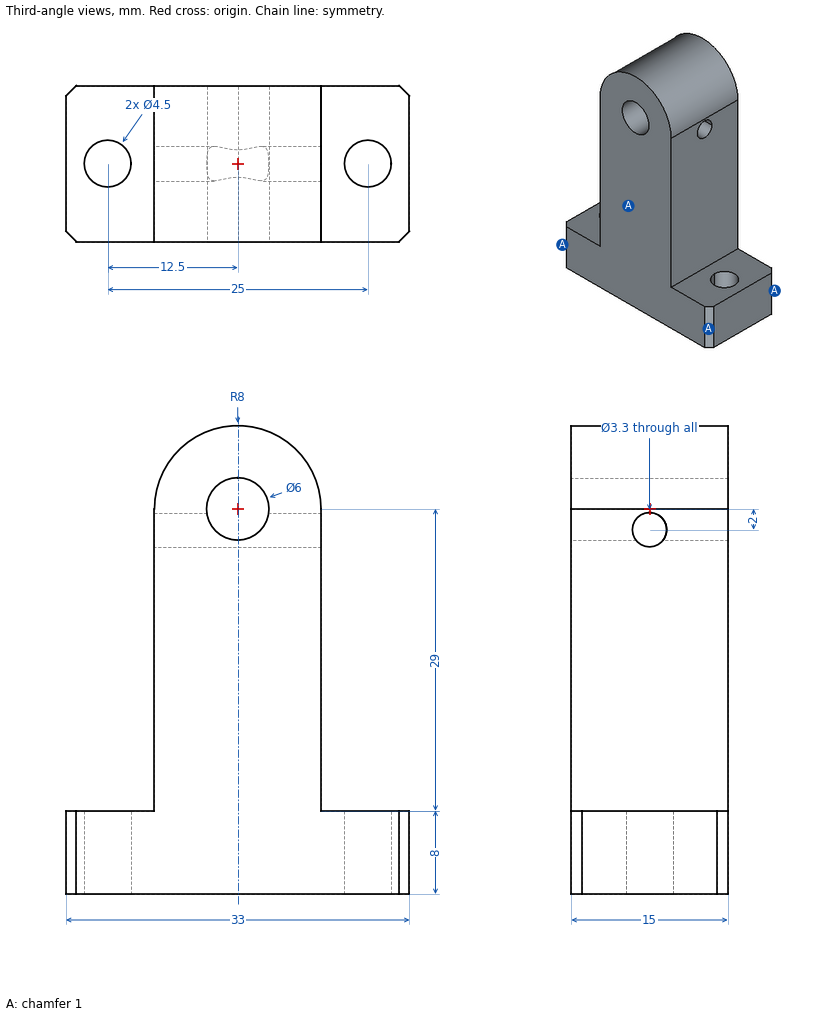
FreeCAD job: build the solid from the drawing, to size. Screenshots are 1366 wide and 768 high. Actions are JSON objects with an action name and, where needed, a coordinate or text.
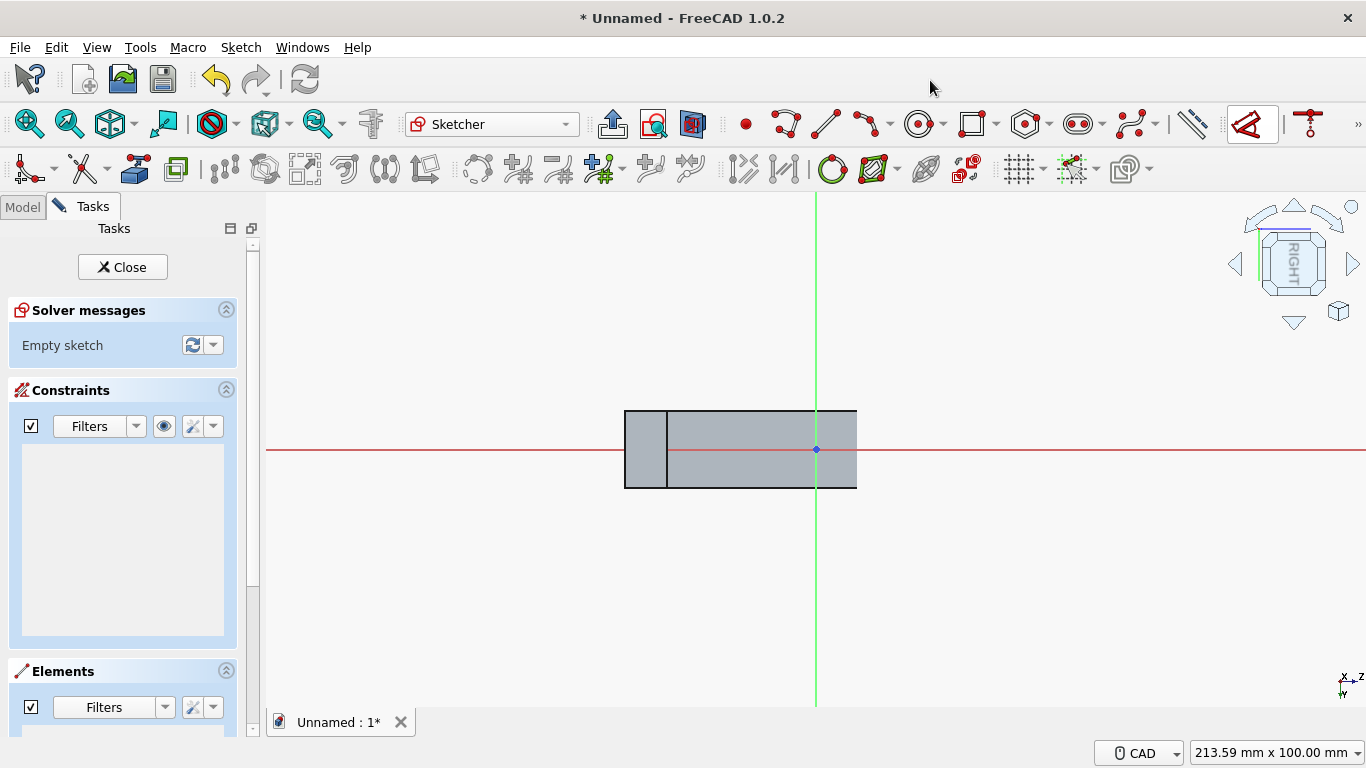
{"action": "left_click", "coordinate": [694, 124]}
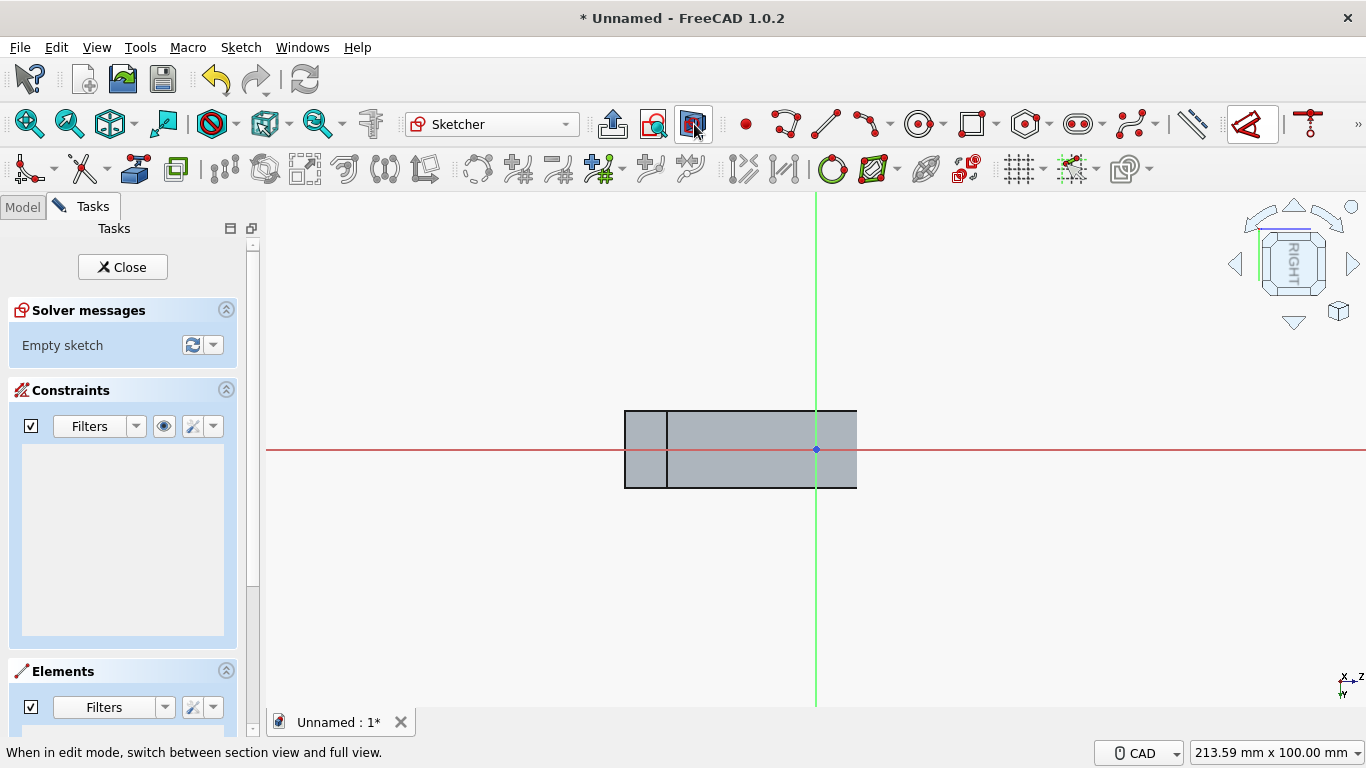
{"action": "scroll", "coordinate": [810, 450], "scroll_direction": "up", "scroll_amount": 15}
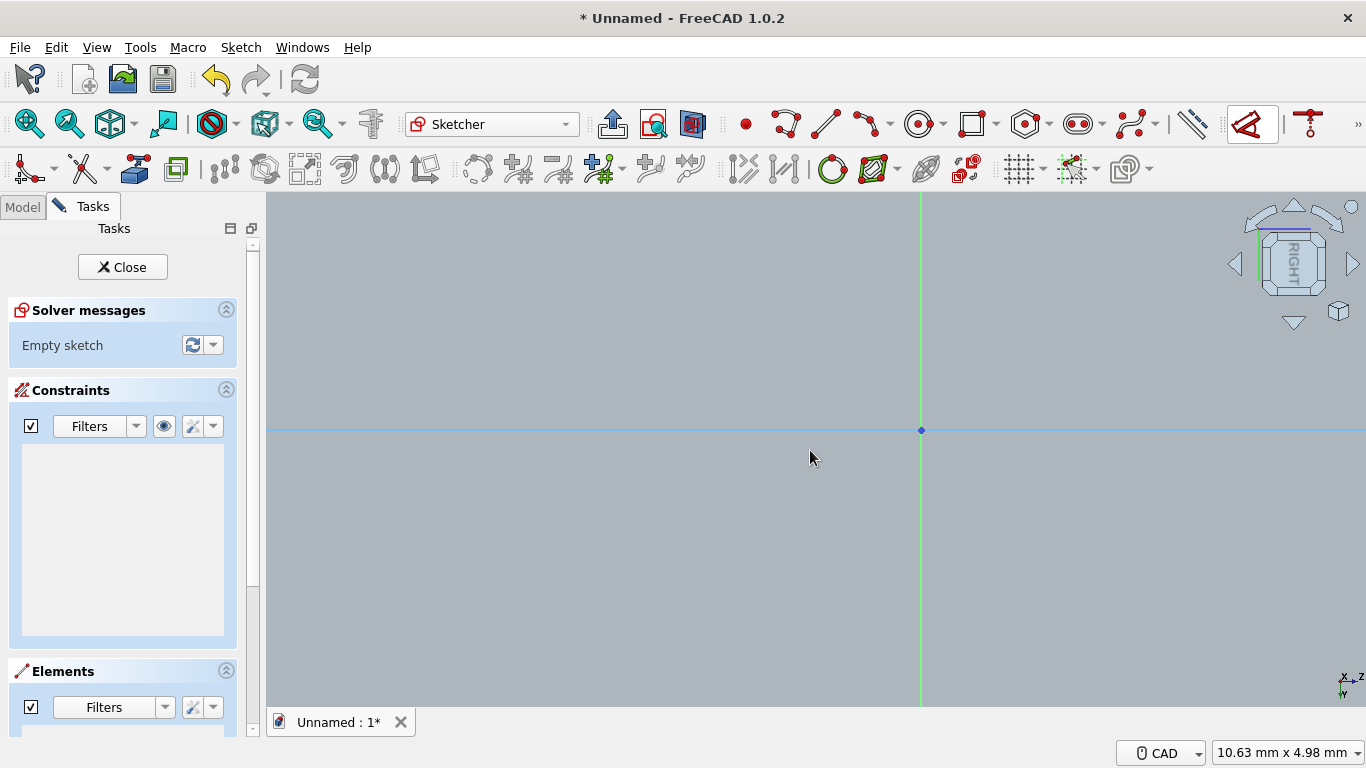
{"action": "key", "text": "g c"}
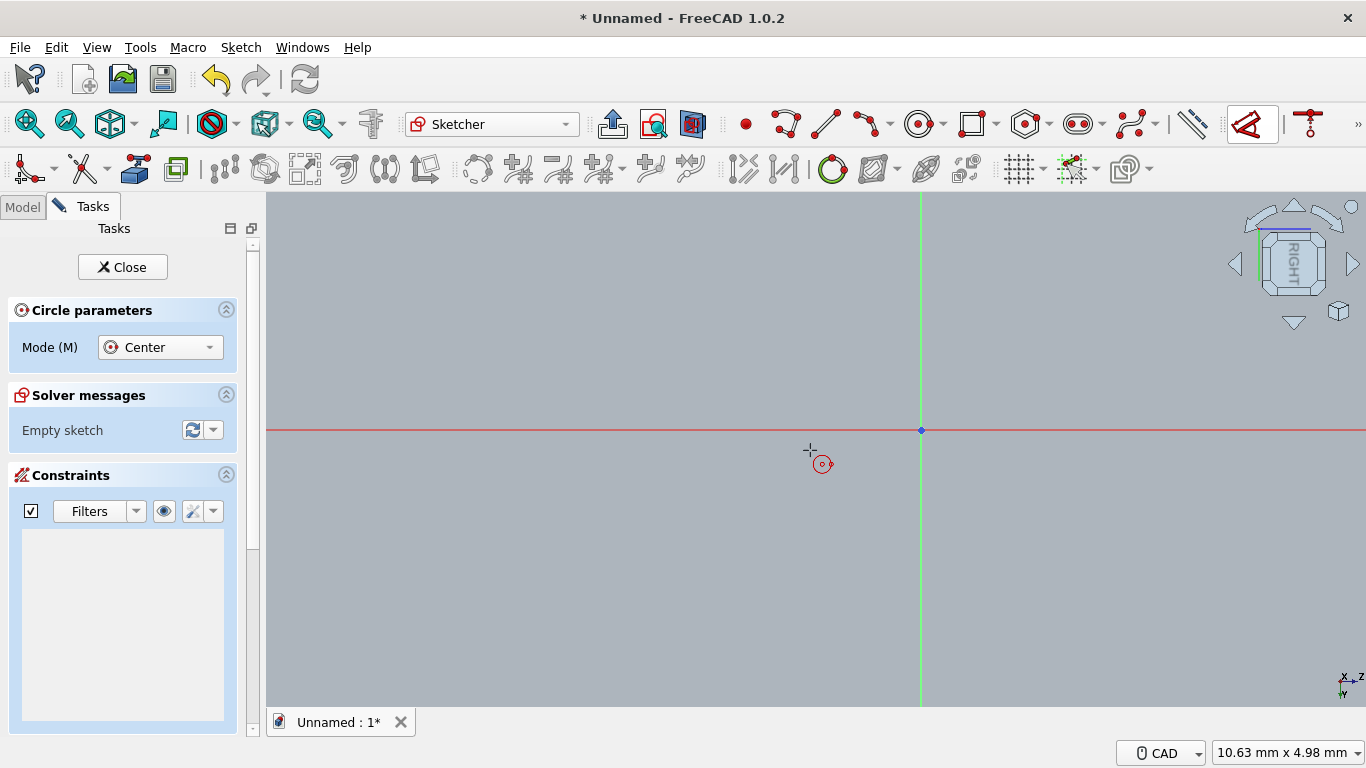
{"action": "left_click", "coordinate": [714, 430]}
{"action": "mouse_move", "coordinate": [835, 310]}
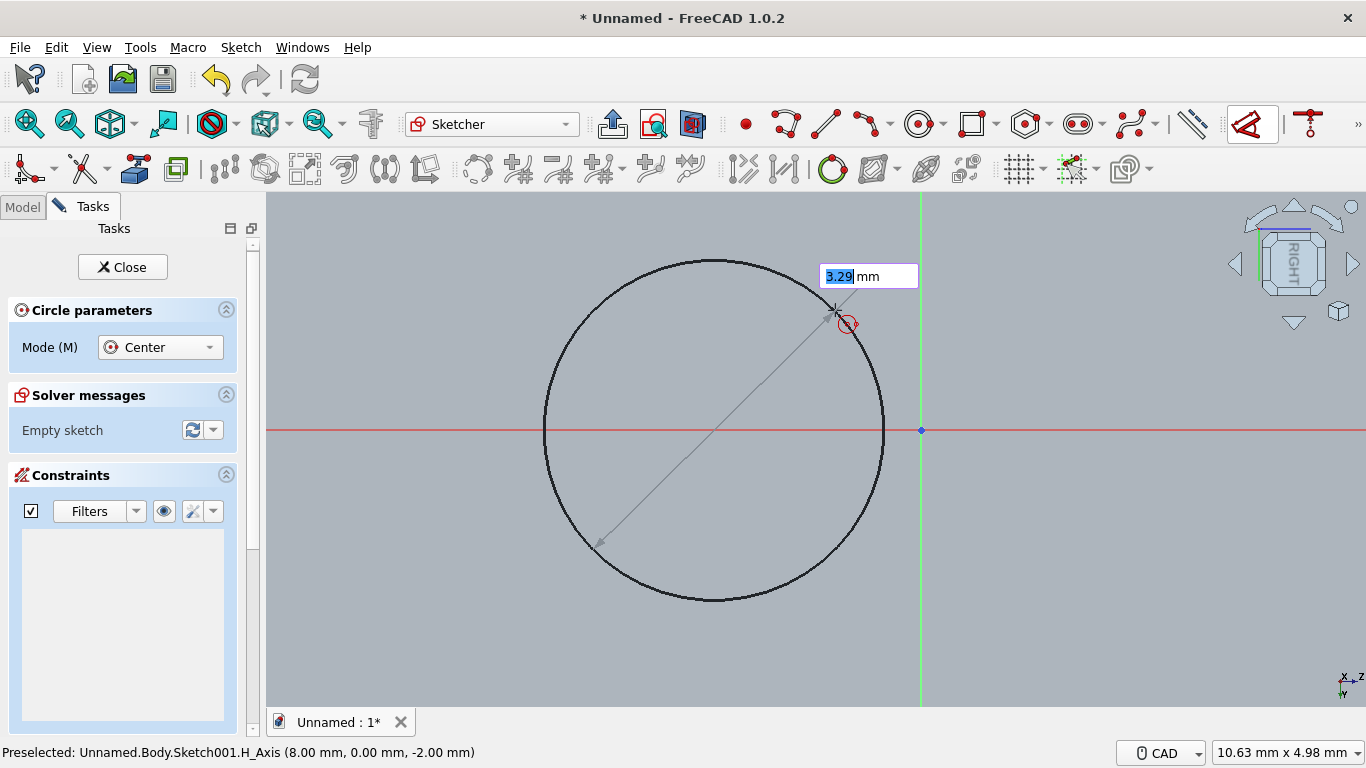
{"action": "type", "text": "3.3"}
{"action": "key", "text": "Return"}
{"action": "key", "text": "Escape"}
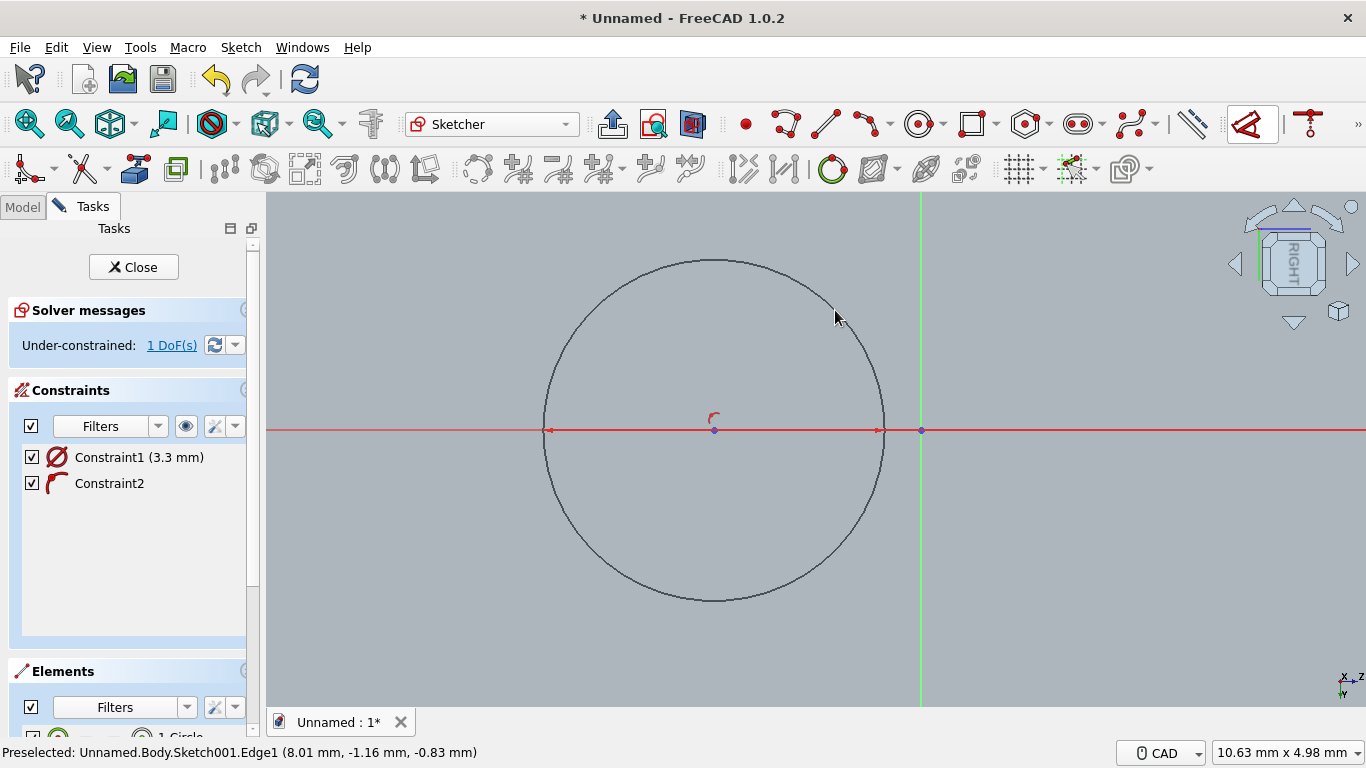
{"action": "key", "text": "d"}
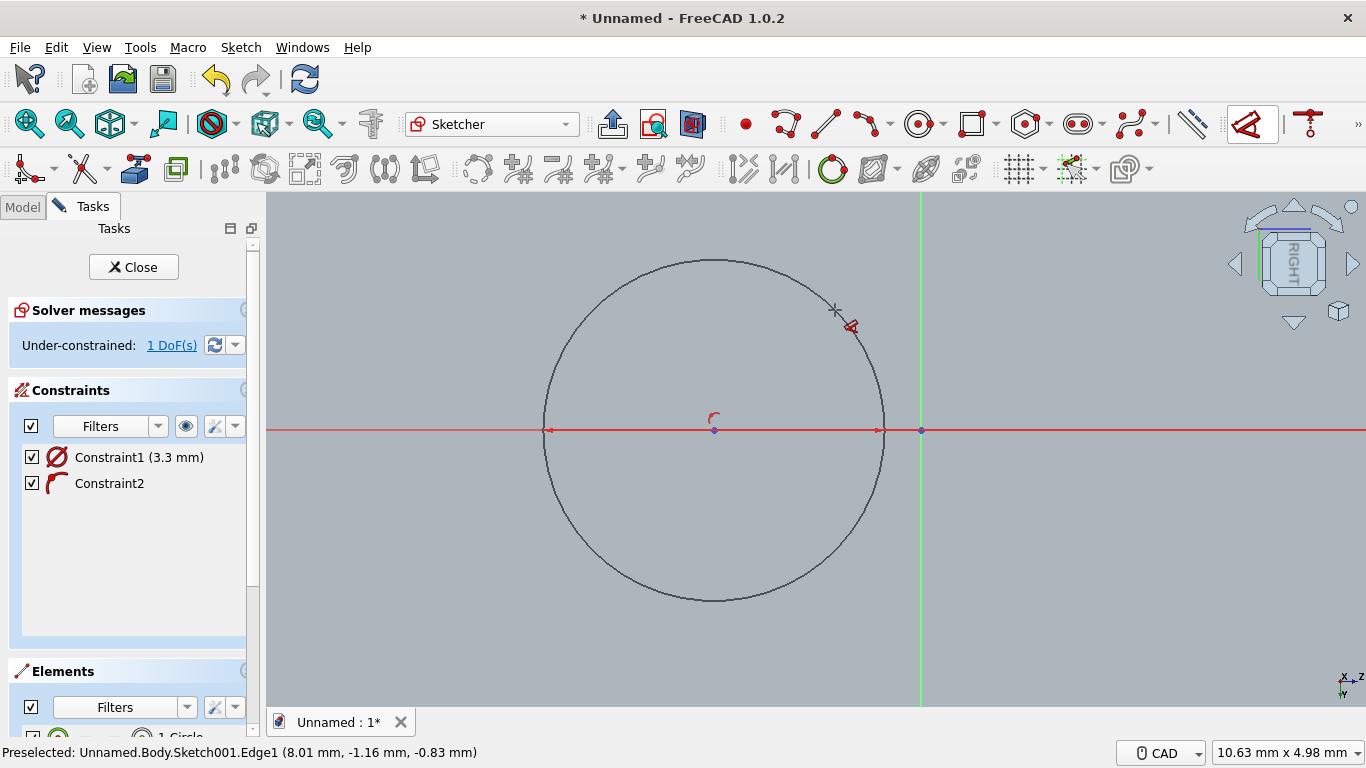
{"action": "left_click", "coordinate": [714, 430]}
{"action": "left_click", "coordinate": [818, 464]}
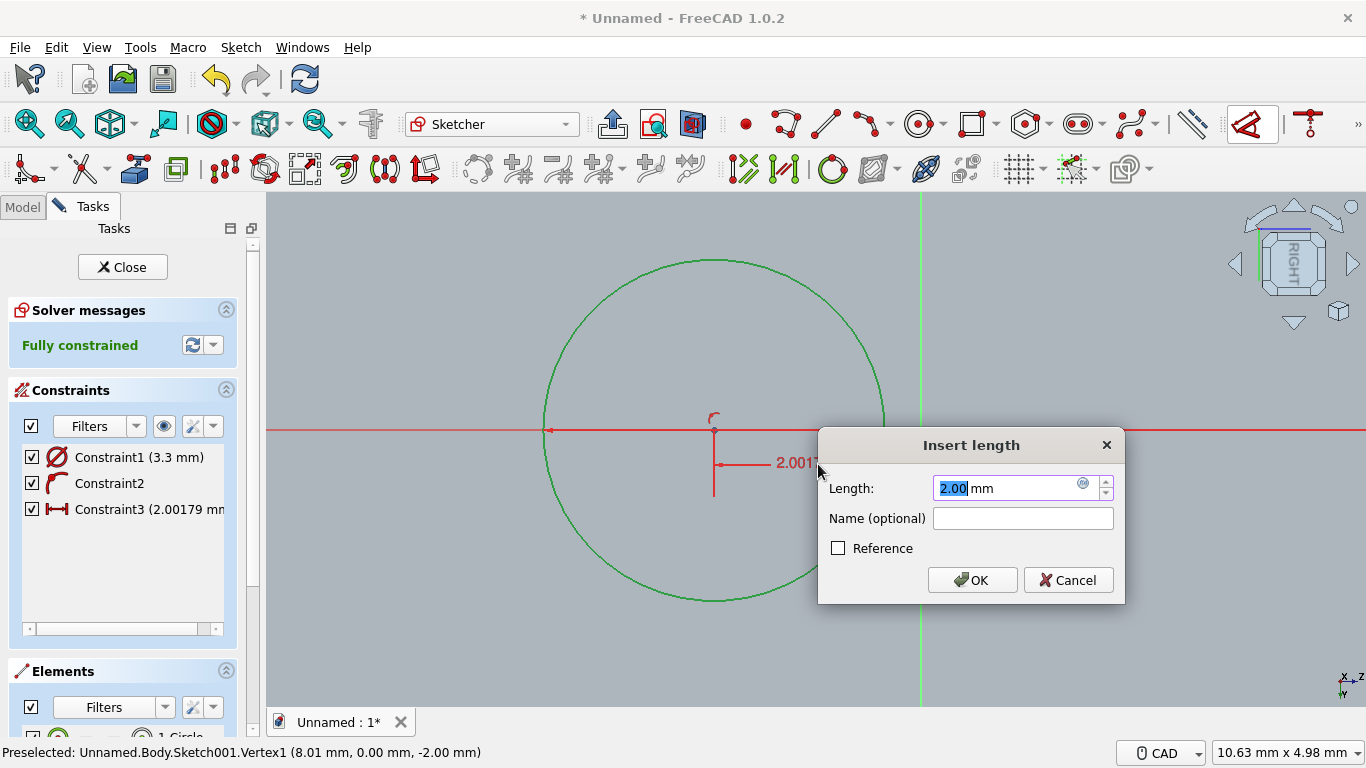
{"action": "type", "text": "2"}
{"action": "key", "text": "Return"}
{"action": "key", "text": "Escape"}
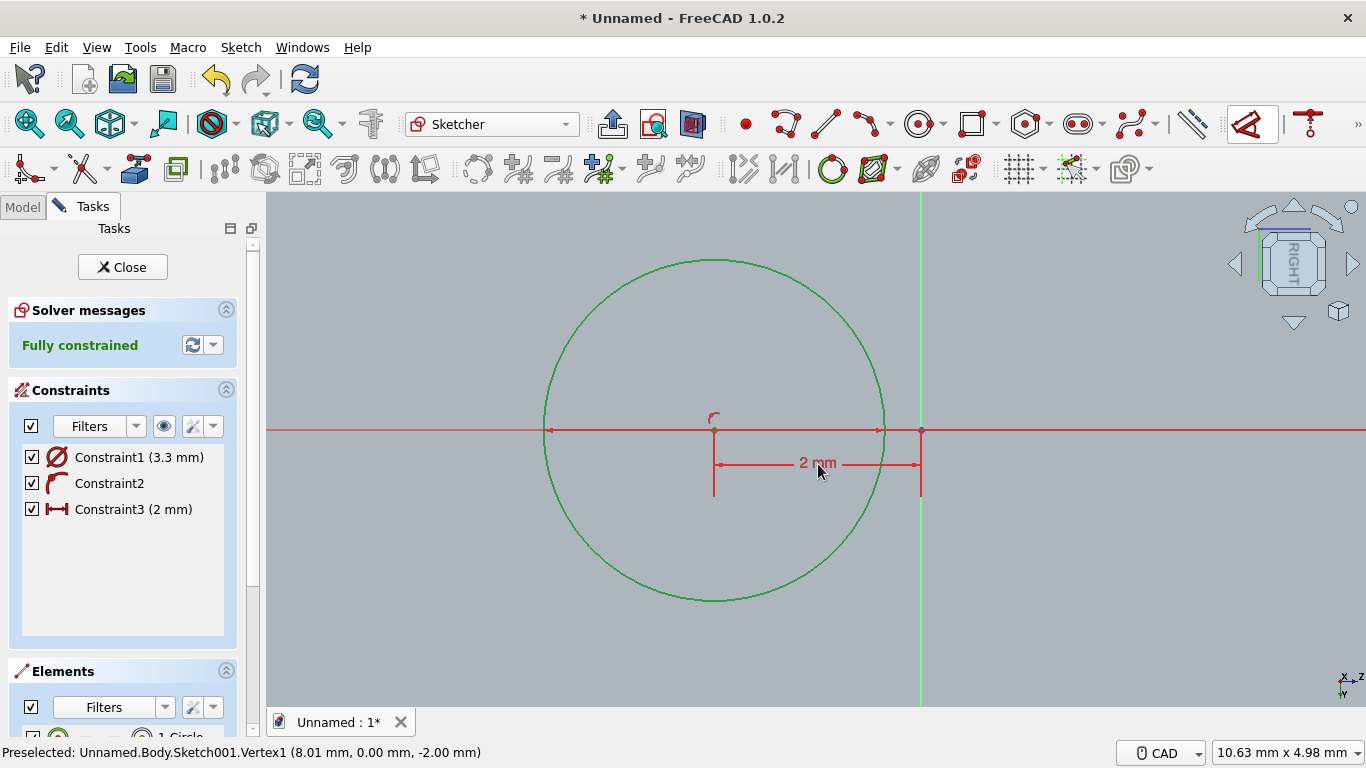
{"action": "left_click", "coordinate": [123, 267]}